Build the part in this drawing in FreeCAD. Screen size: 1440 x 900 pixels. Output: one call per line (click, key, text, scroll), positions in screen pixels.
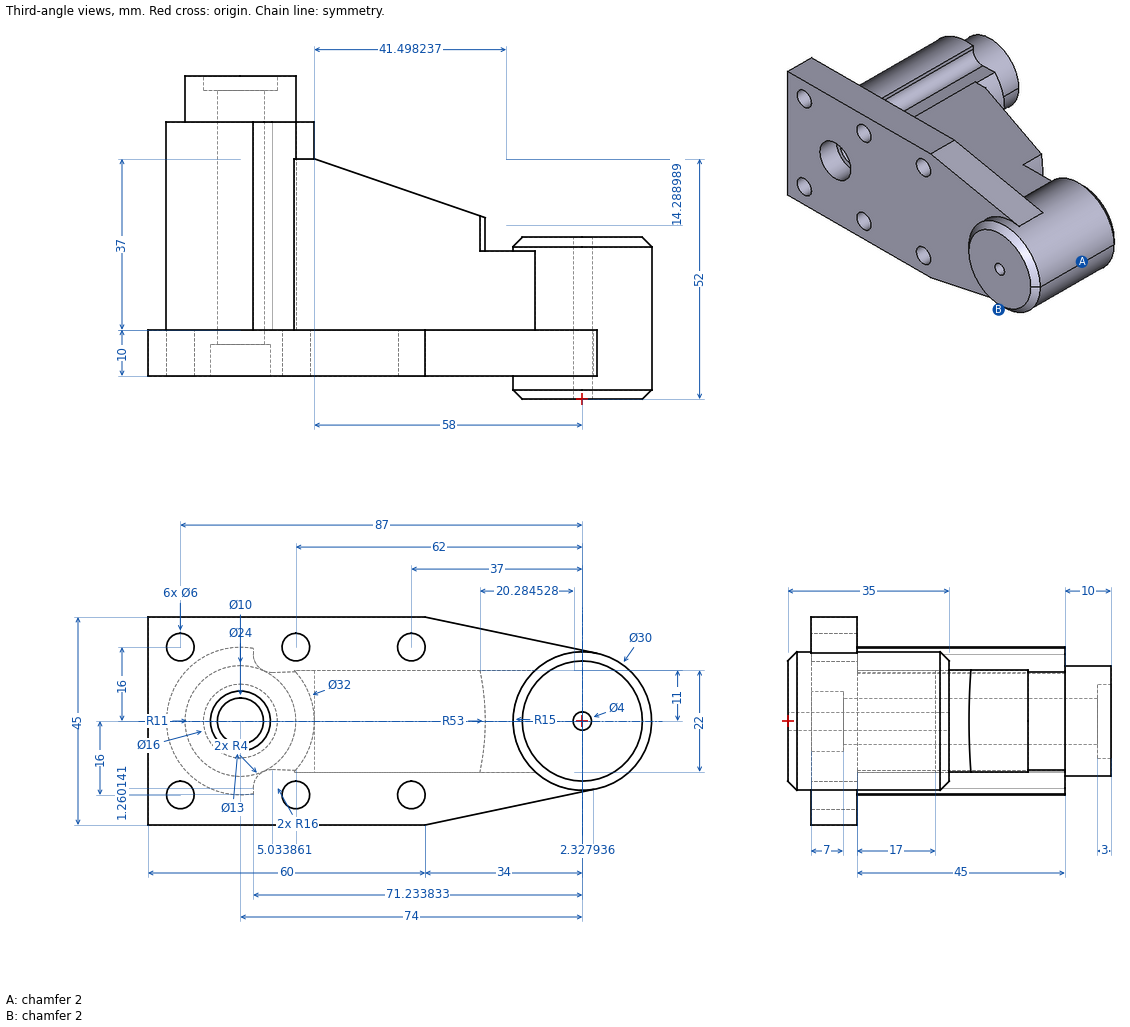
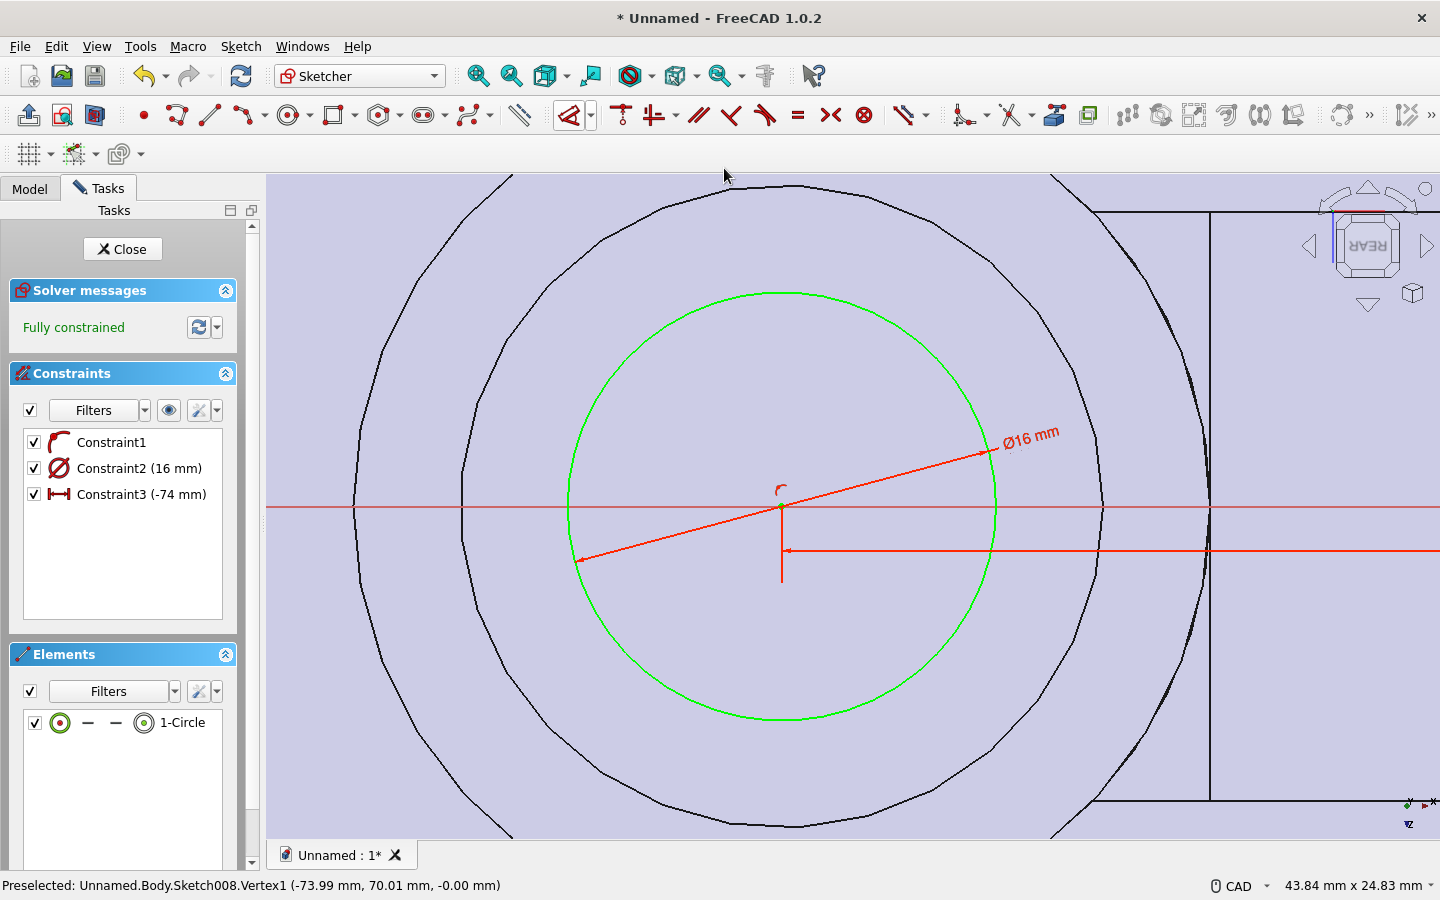
click(123, 249)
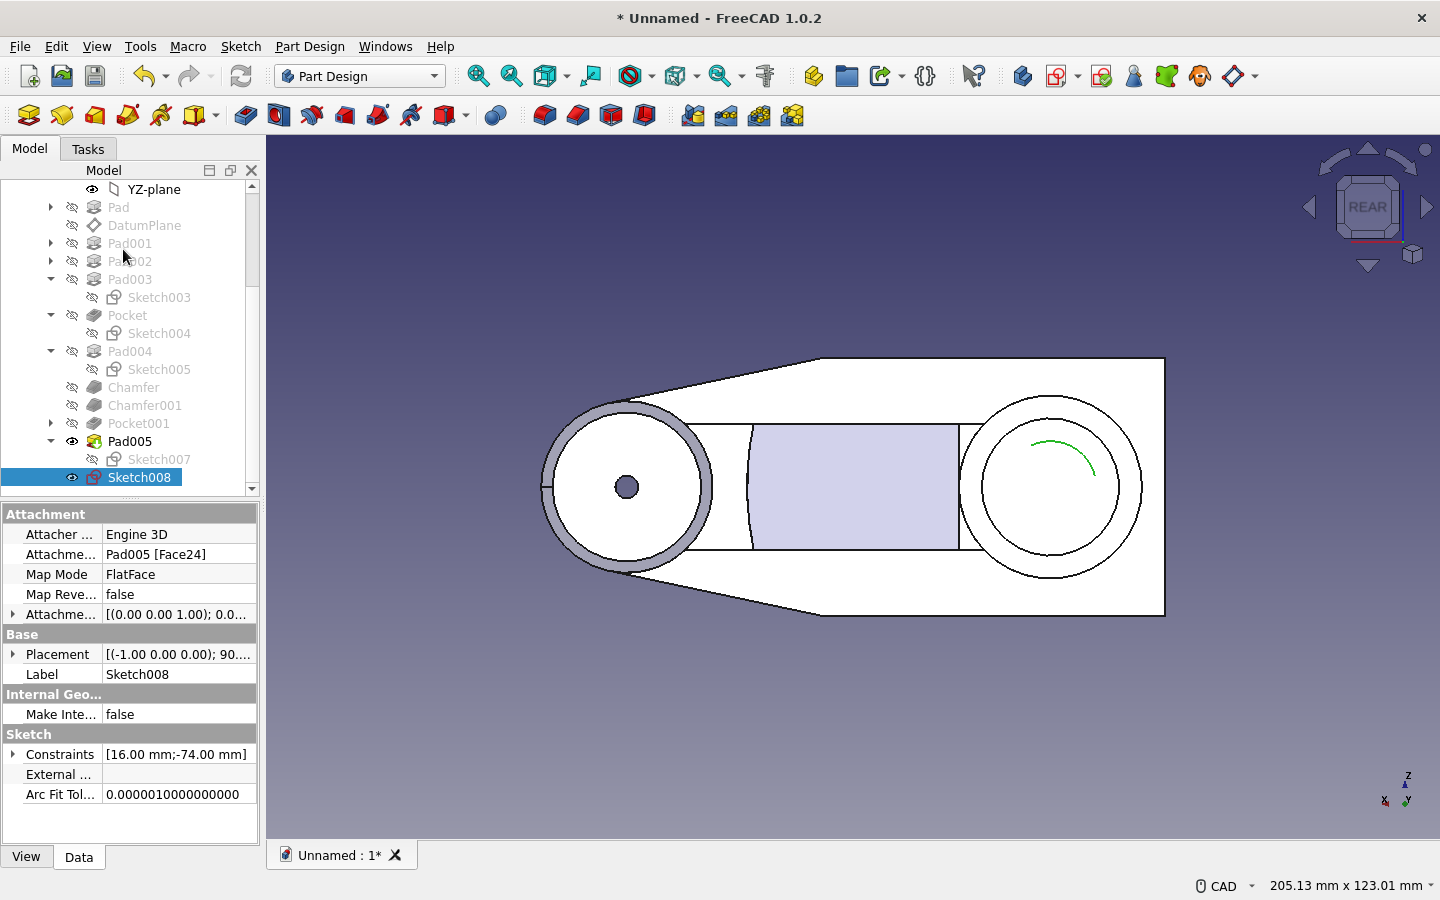
click(246, 116)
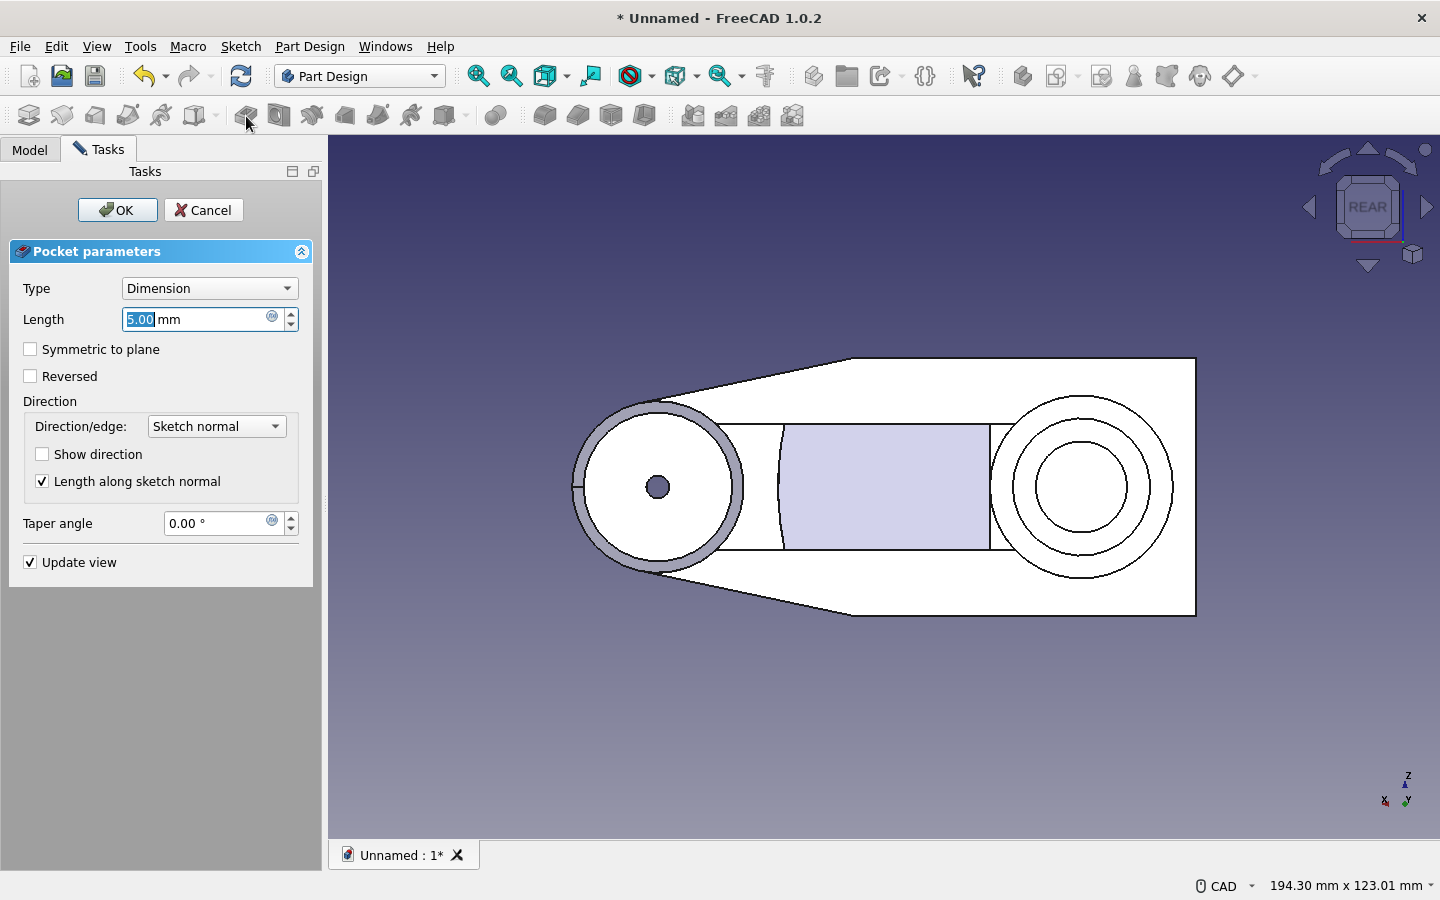
text(3)
key(Tab)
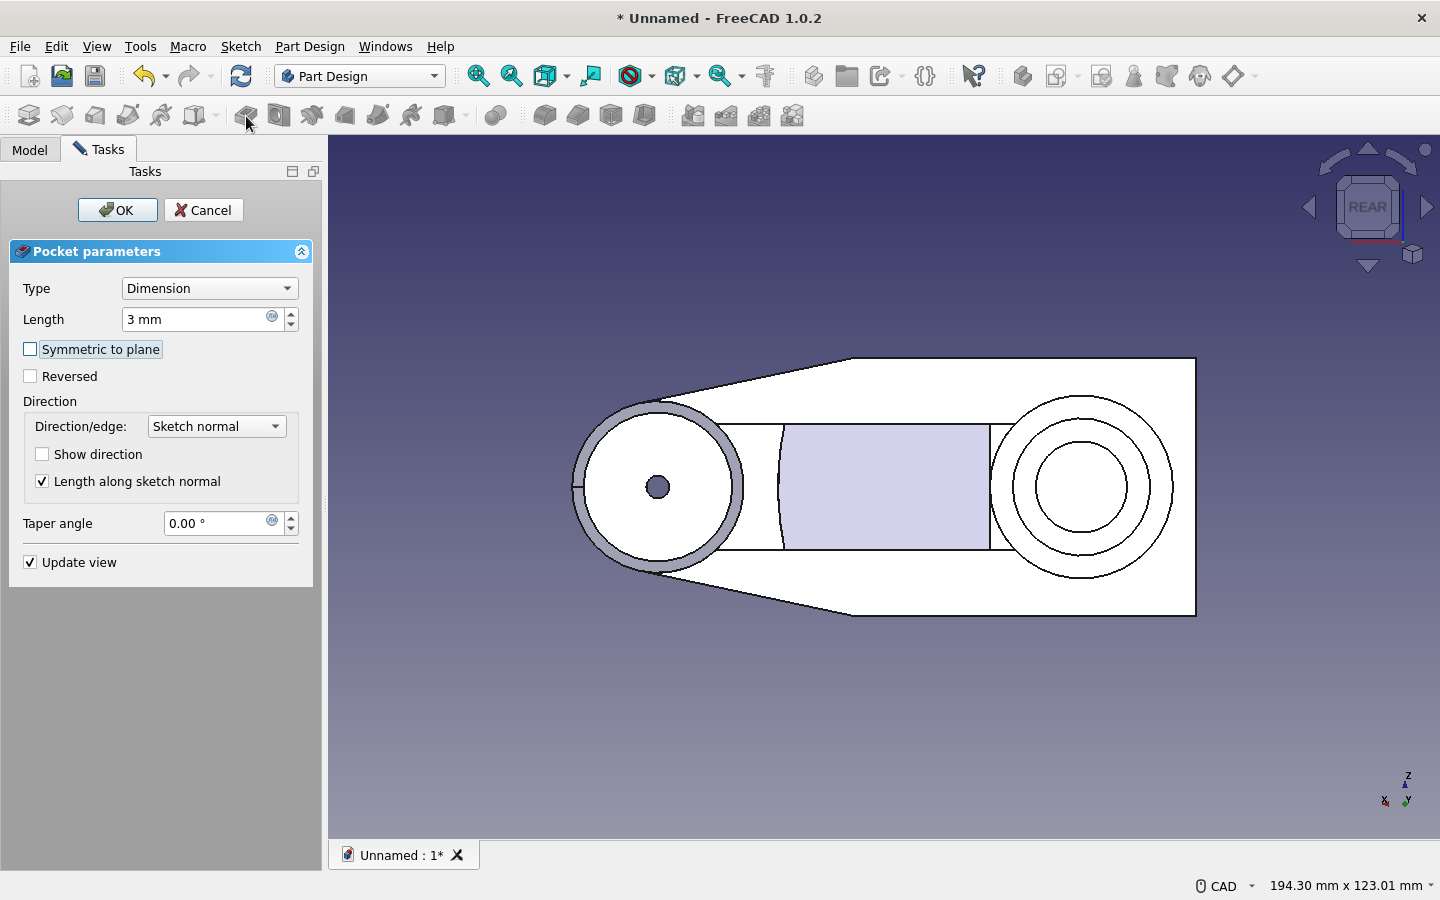
click(118, 210)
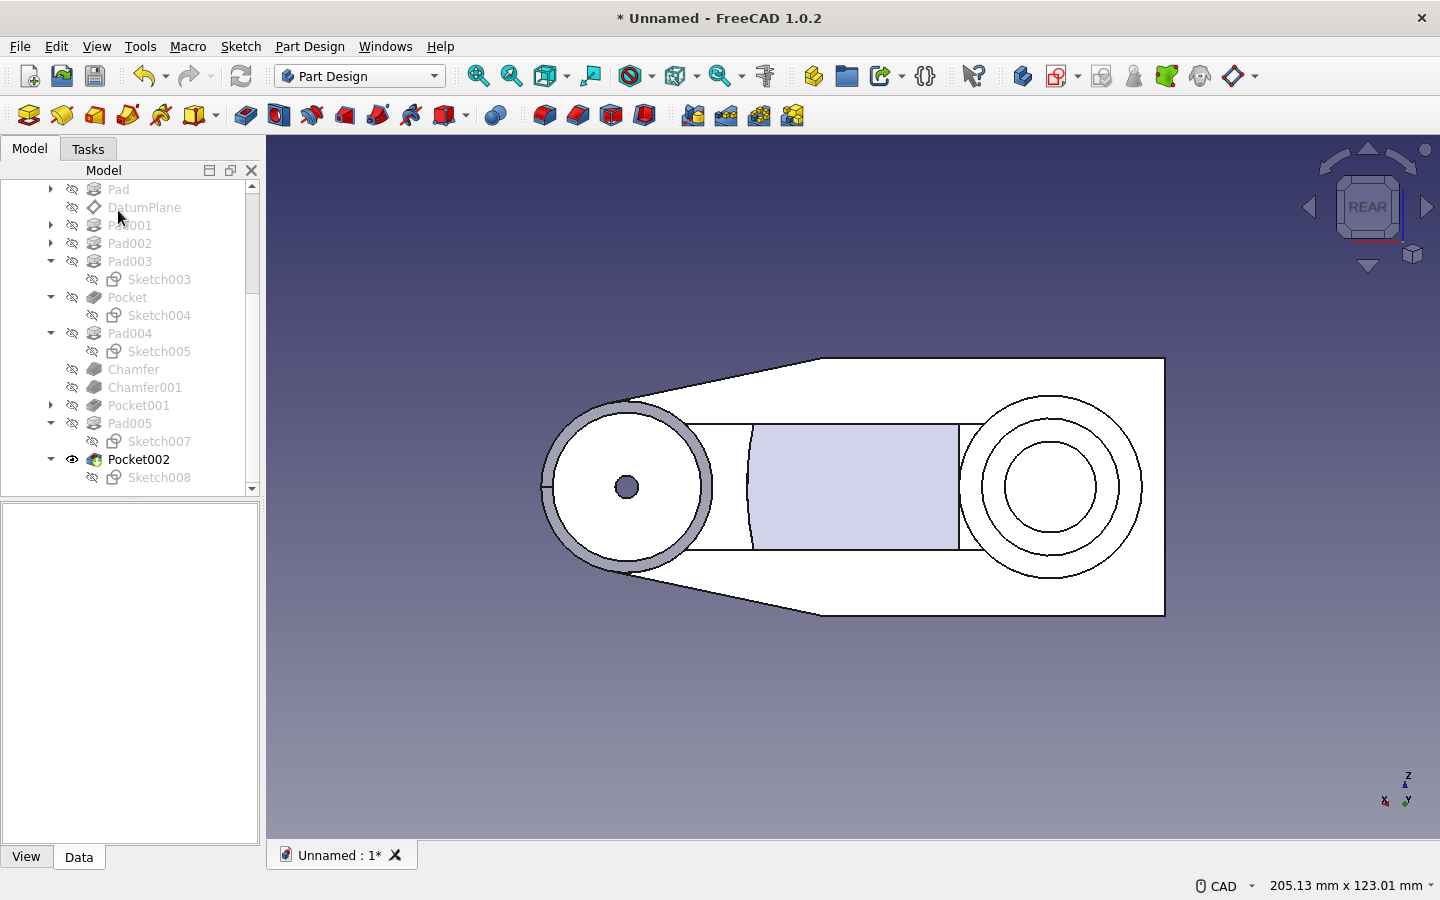
click(1050, 486)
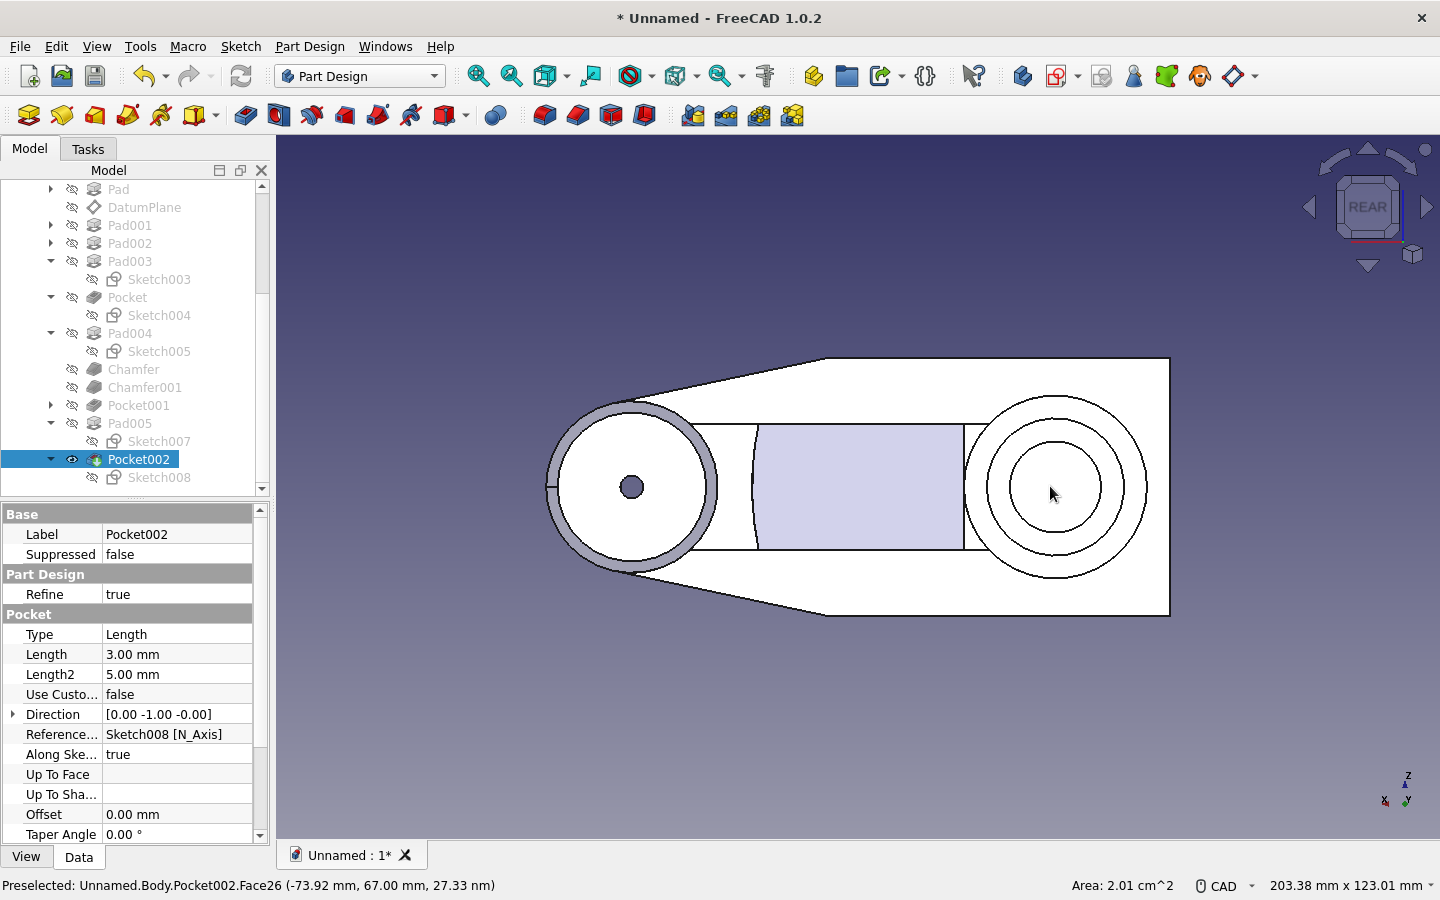
click(1056, 76)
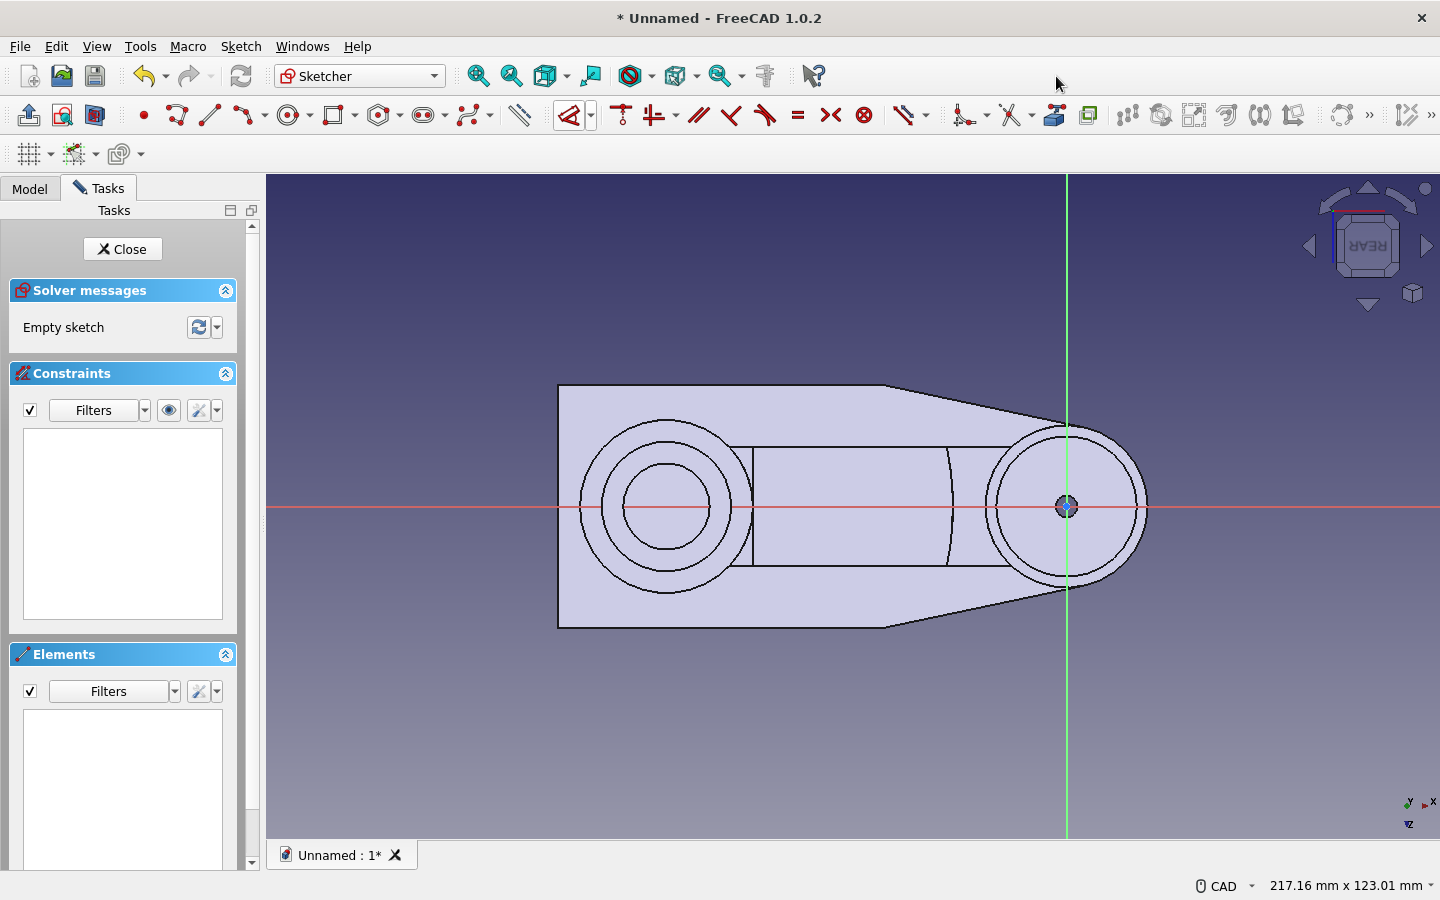
scroll(648, 506, up, 10)